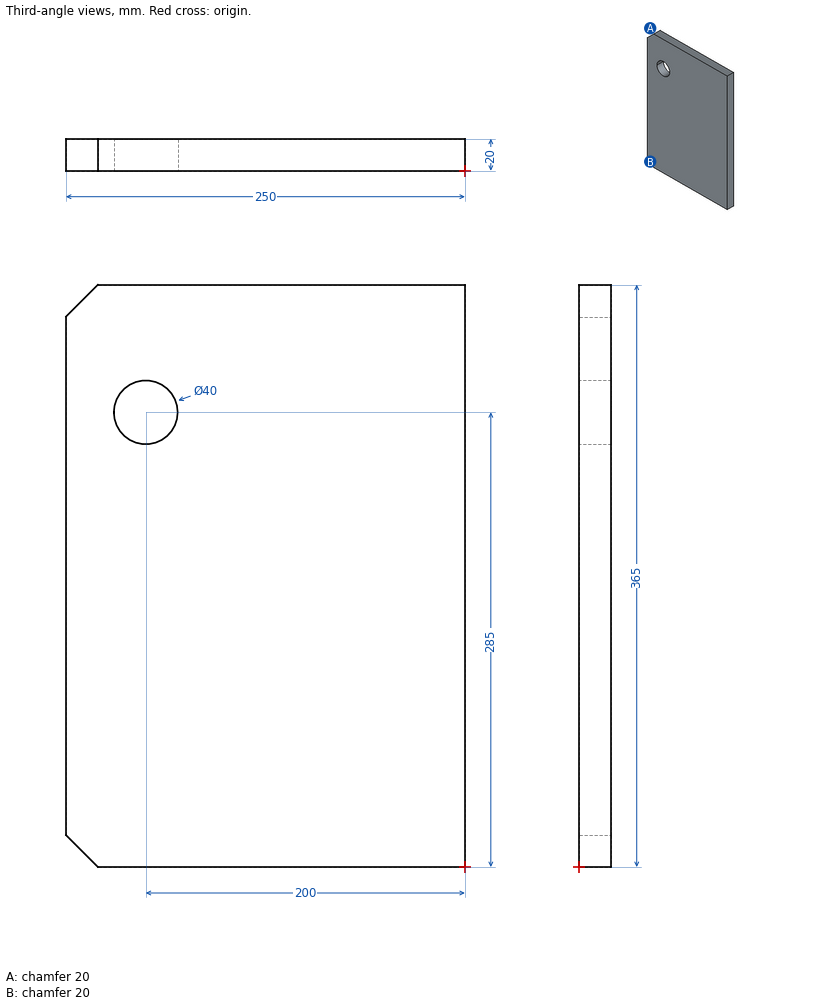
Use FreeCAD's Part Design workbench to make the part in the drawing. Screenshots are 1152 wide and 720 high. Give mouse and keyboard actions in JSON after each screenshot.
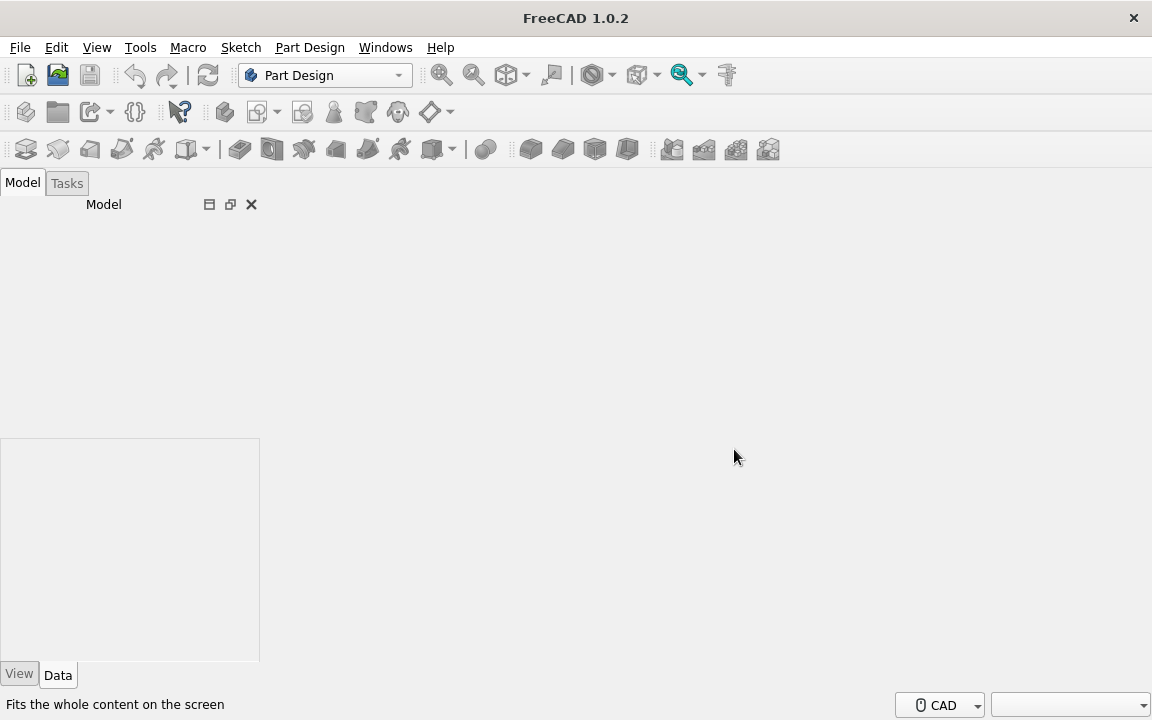
{"action": "key", "text": "ctrl+n"}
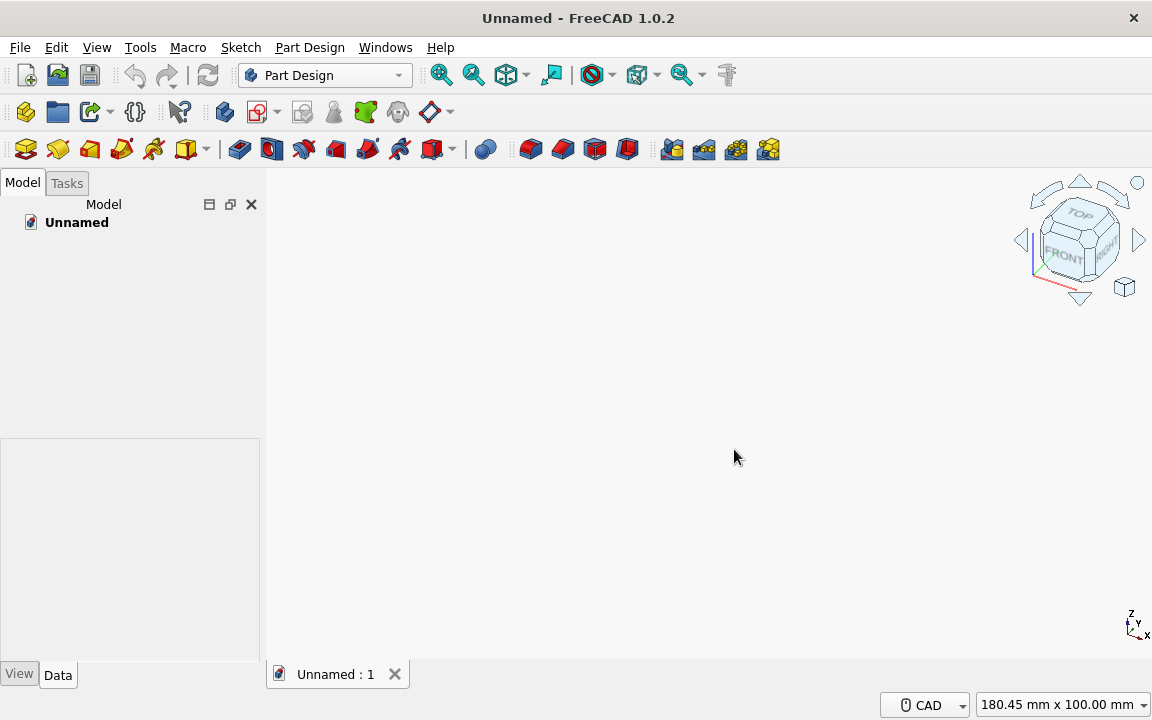
{"action": "left_click", "coordinate": [258, 112]}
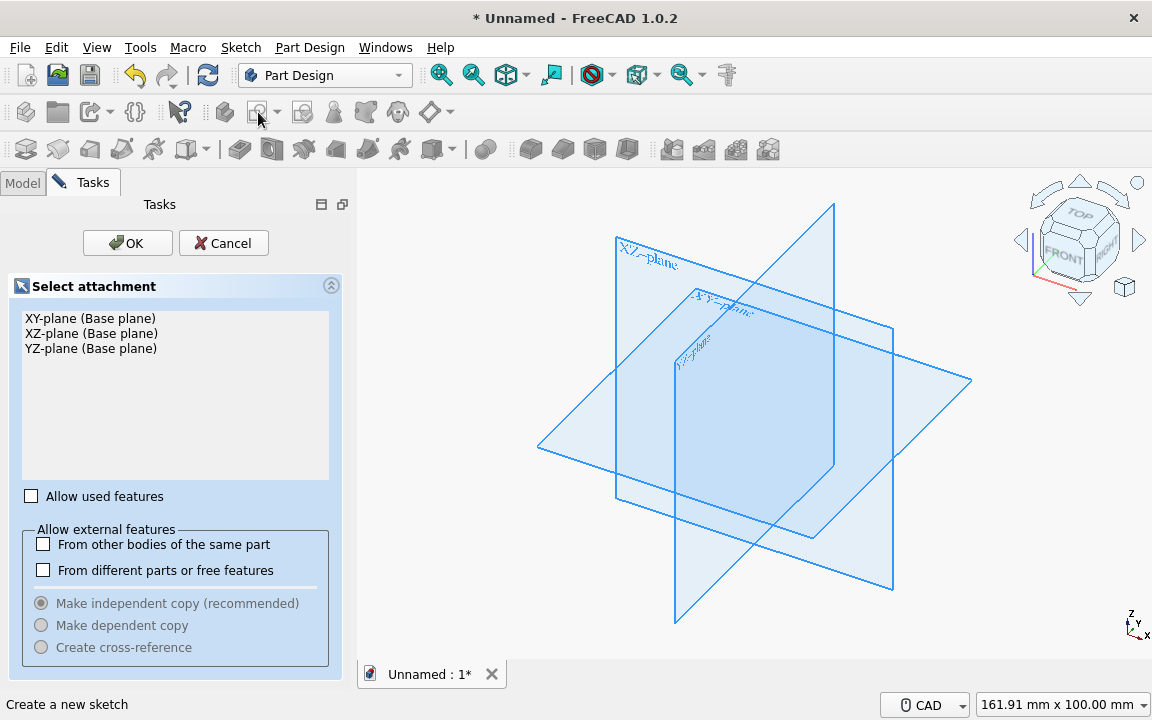
{"action": "left_click", "coordinate": [82, 318]}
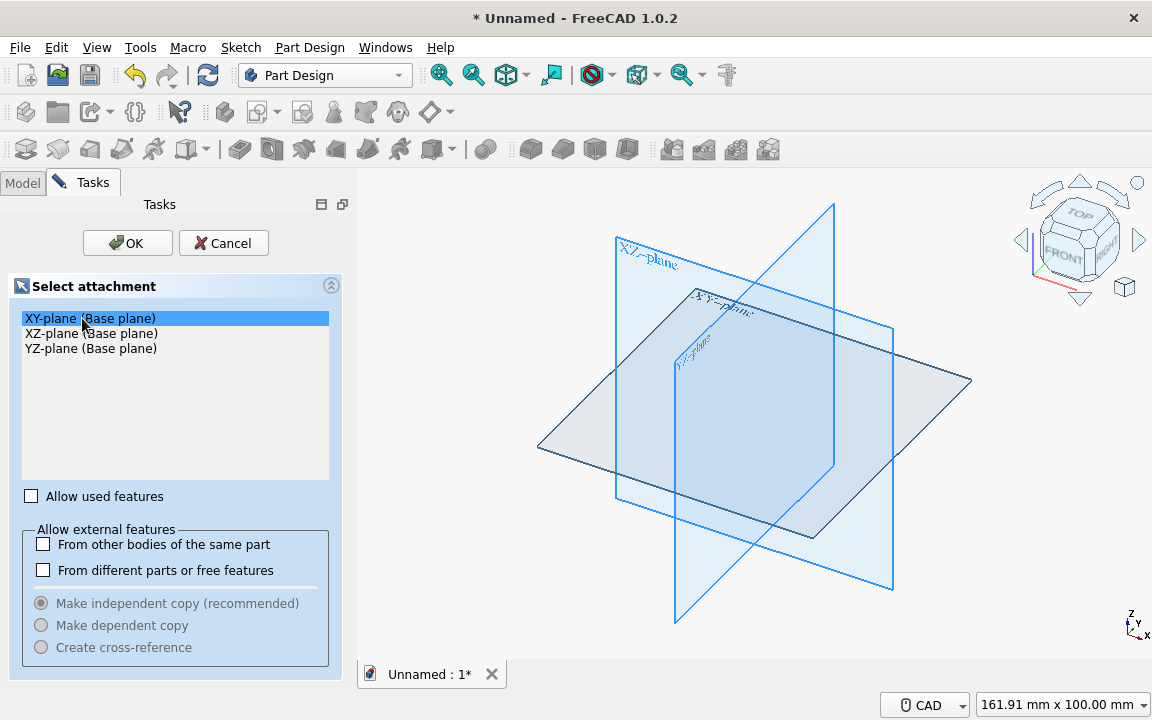
{"action": "left_click", "coordinate": [128, 243]}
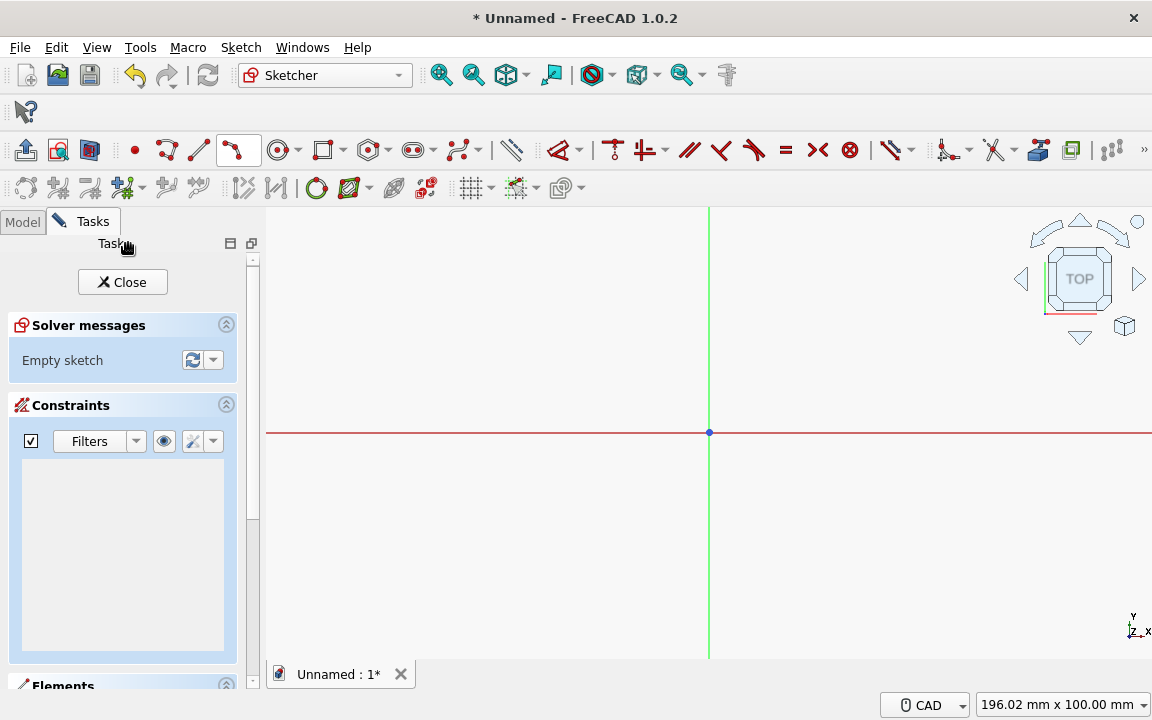
{"action": "scroll", "coordinate": [987, 470], "scroll_direction": "down", "scroll_amount": 4}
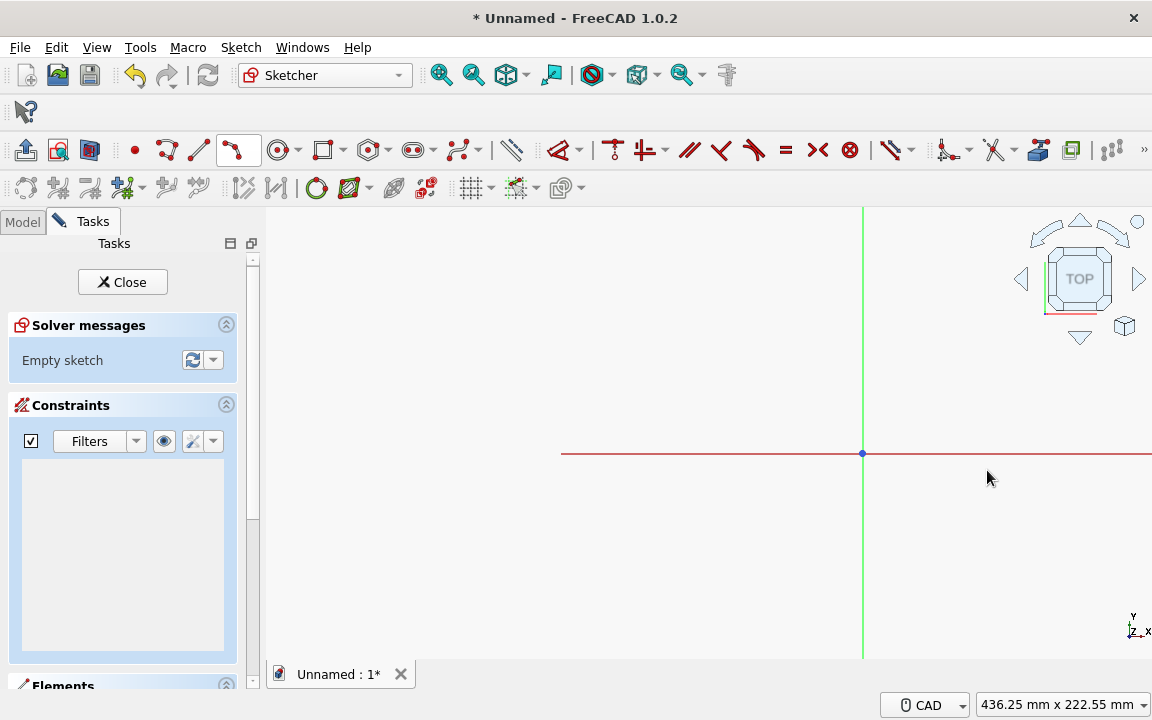
{"action": "key", "text": "g r"}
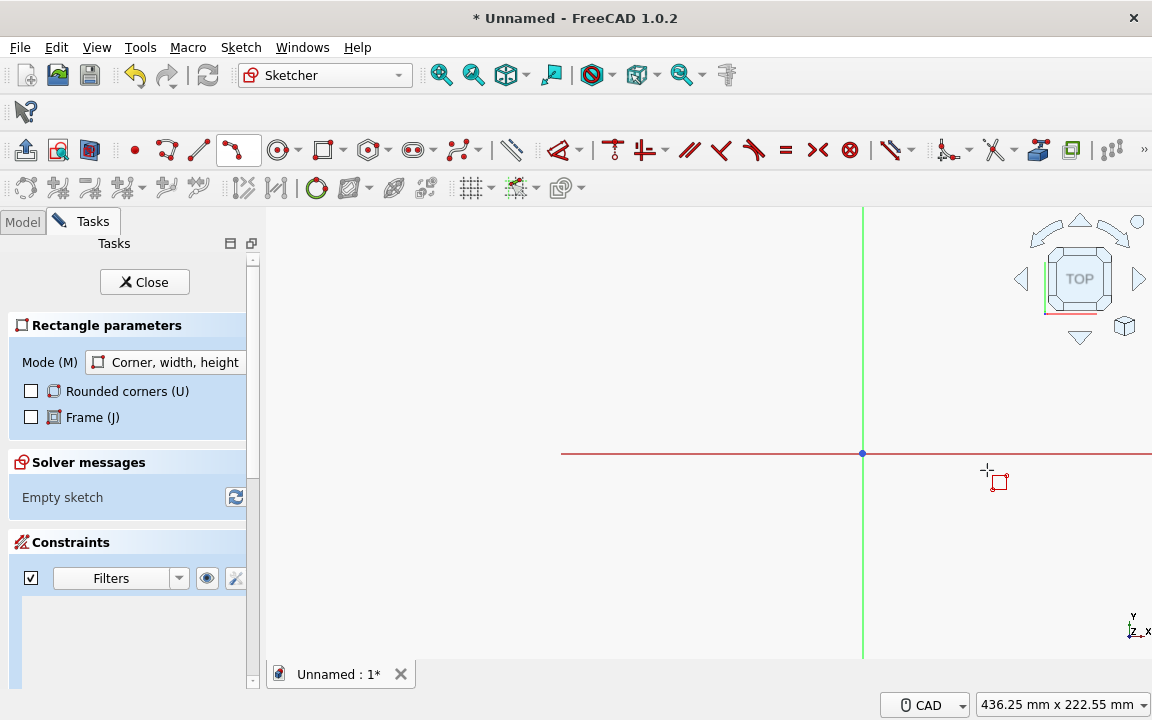
{"action": "left_click", "coordinate": [863, 454]}
{"action": "mouse_move", "coordinate": [355, 413]}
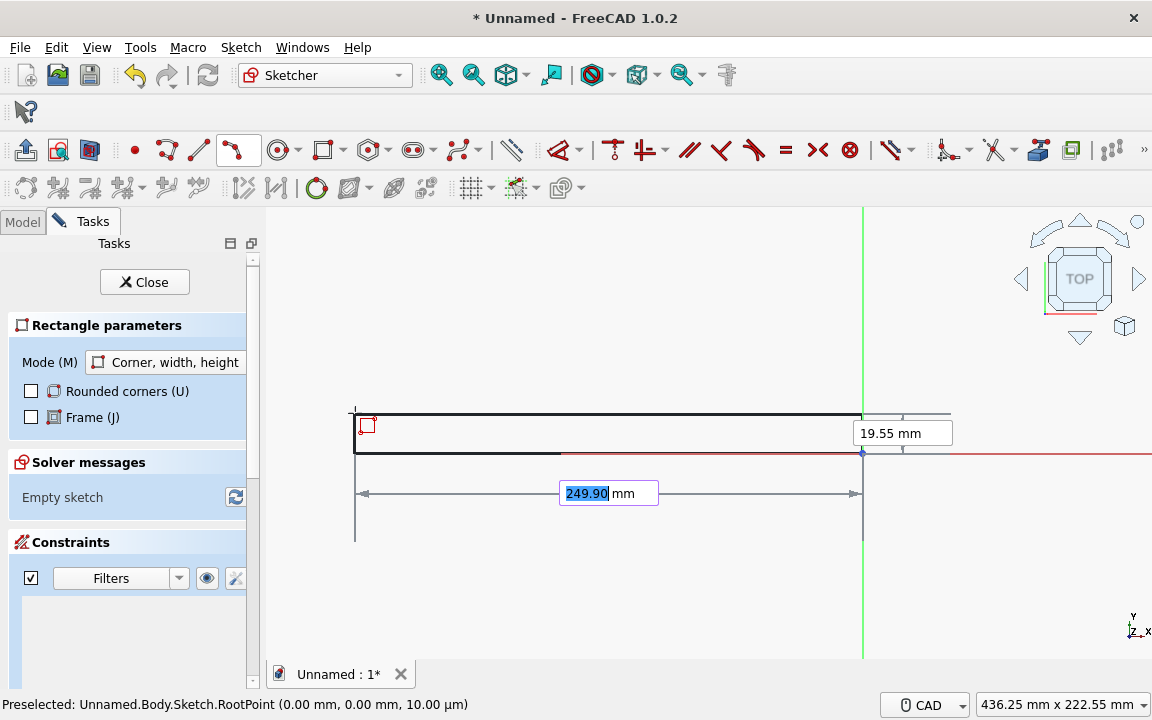
{"action": "type", "text": "250"}
{"action": "key", "text": "Tab"}
{"action": "type", "text": "20"}
{"action": "key", "text": "Return"}
{"action": "key", "text": "Escape"}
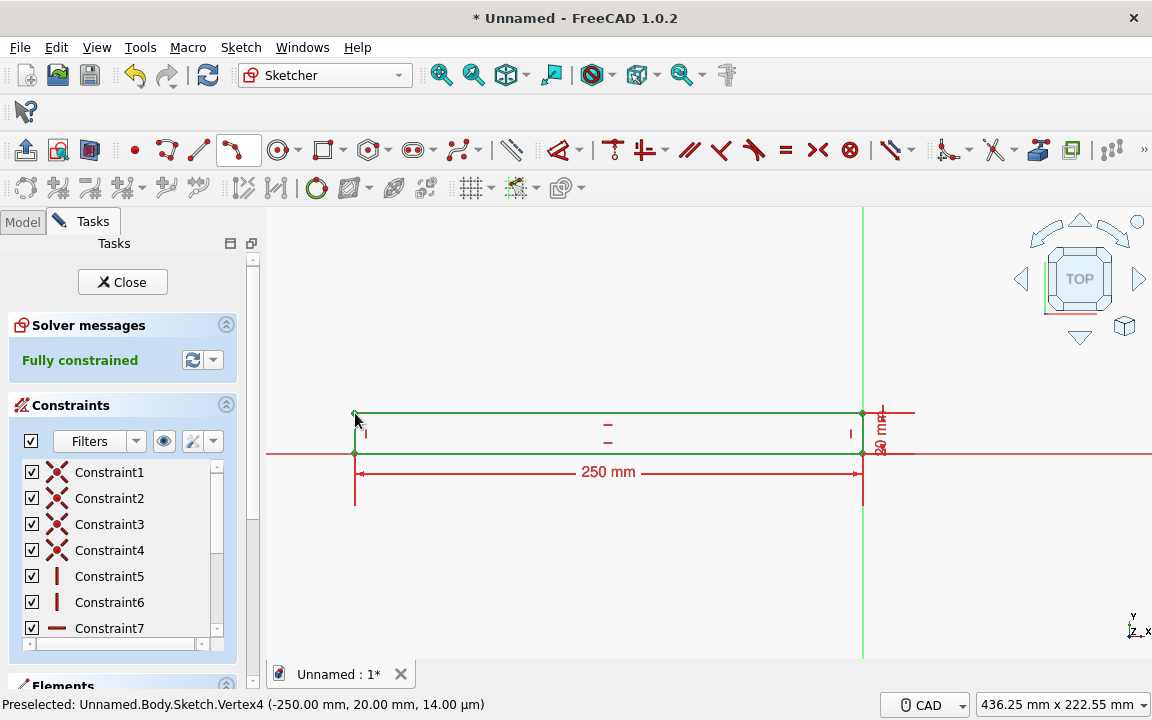
{"action": "left_click", "coordinate": [123, 282]}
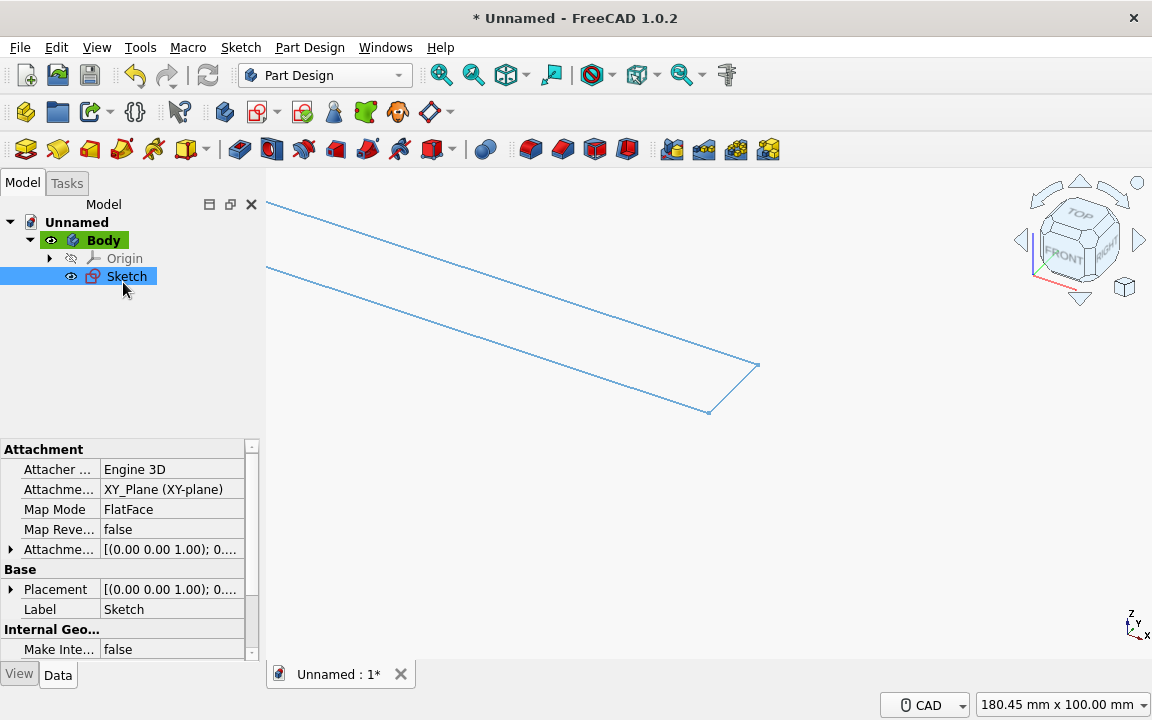
{"action": "left_click", "coordinate": [26, 150]}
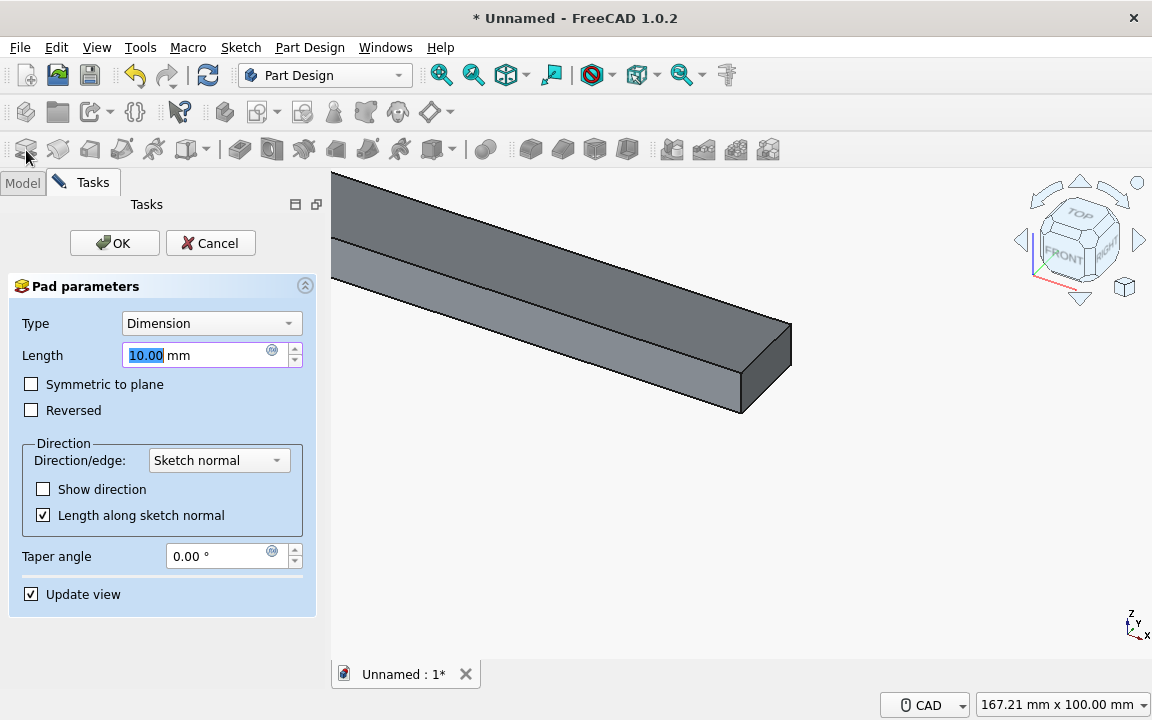
{"action": "type", "text": "365"}
{"action": "key", "text": "Tab"}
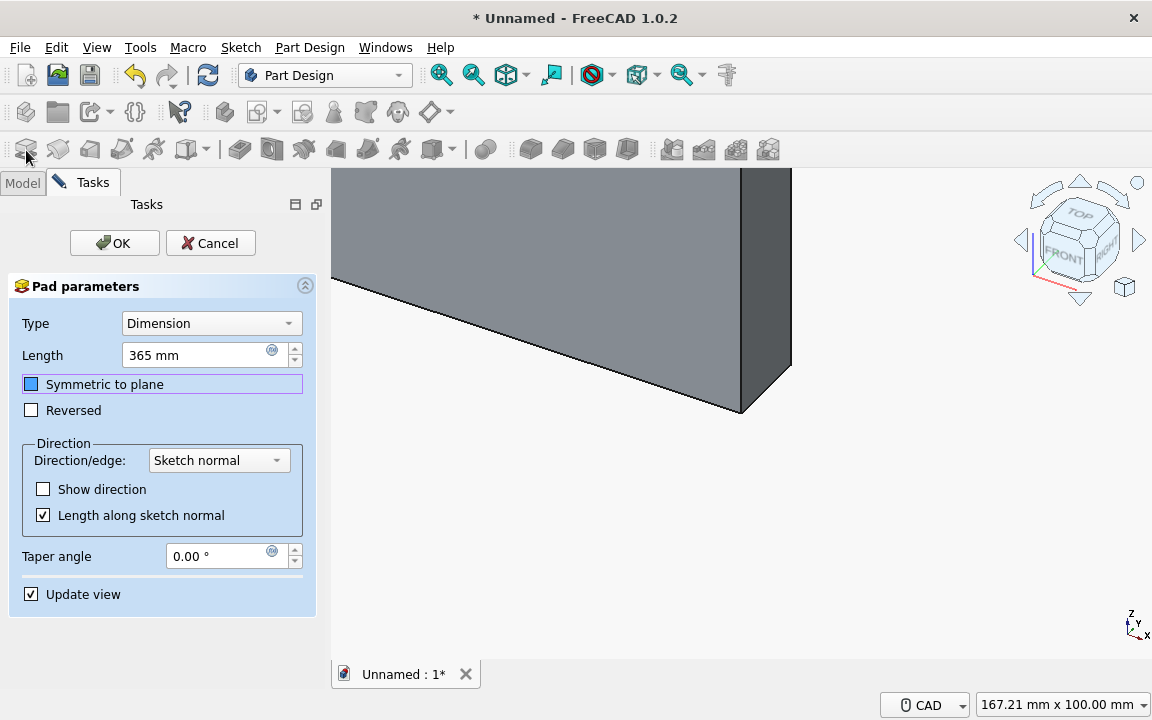
{"action": "left_click", "coordinate": [115, 243]}